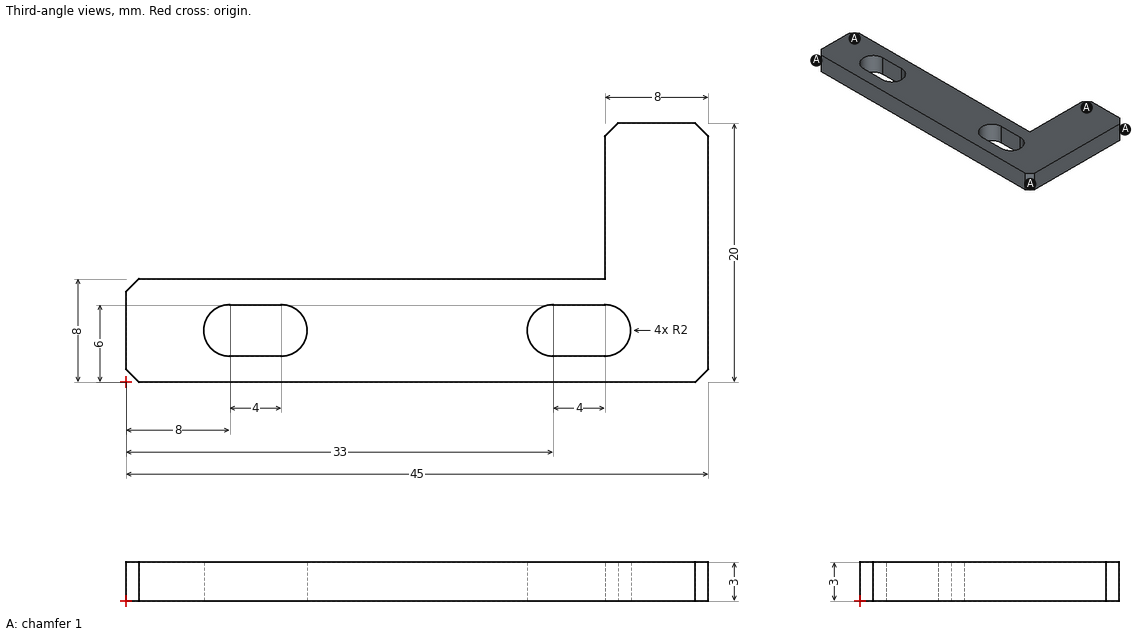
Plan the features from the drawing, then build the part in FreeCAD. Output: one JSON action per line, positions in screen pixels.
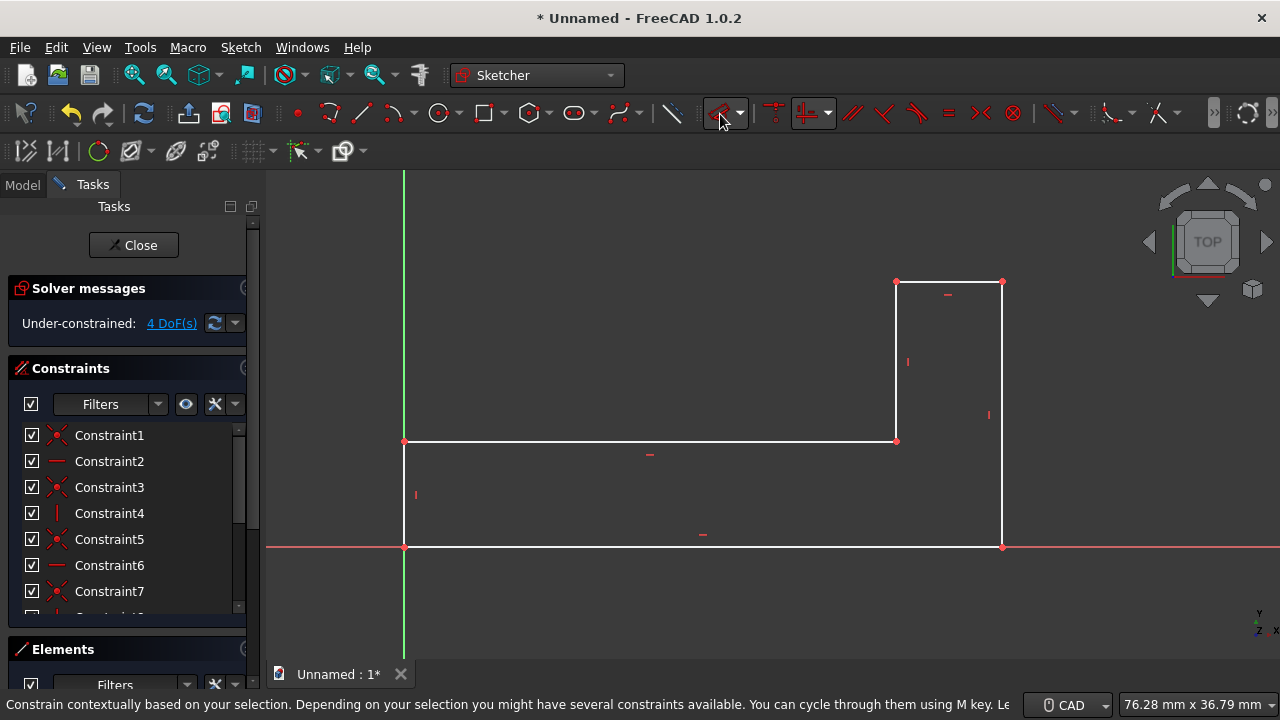
{"action": "left_click", "coordinate": [970, 282]}
{"action": "left_click", "coordinate": [949, 248]}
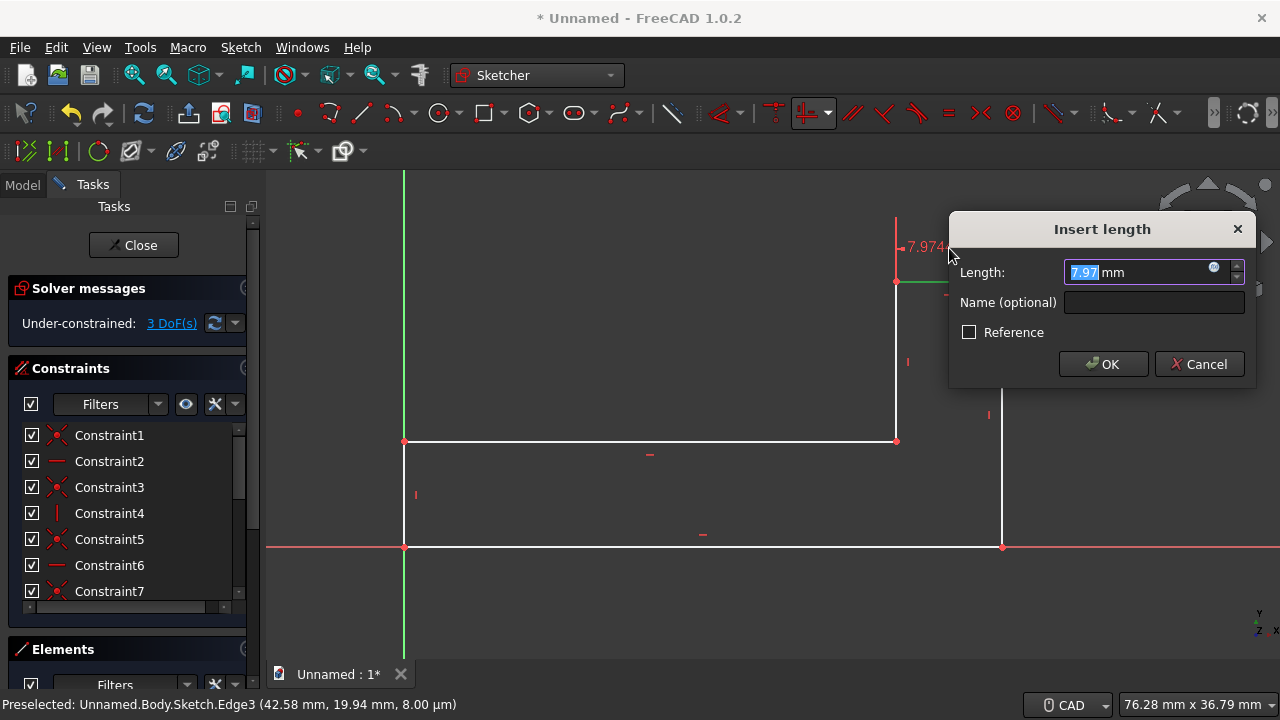
{"action": "type", "text": "8"}
{"action": "key", "text": "Return"}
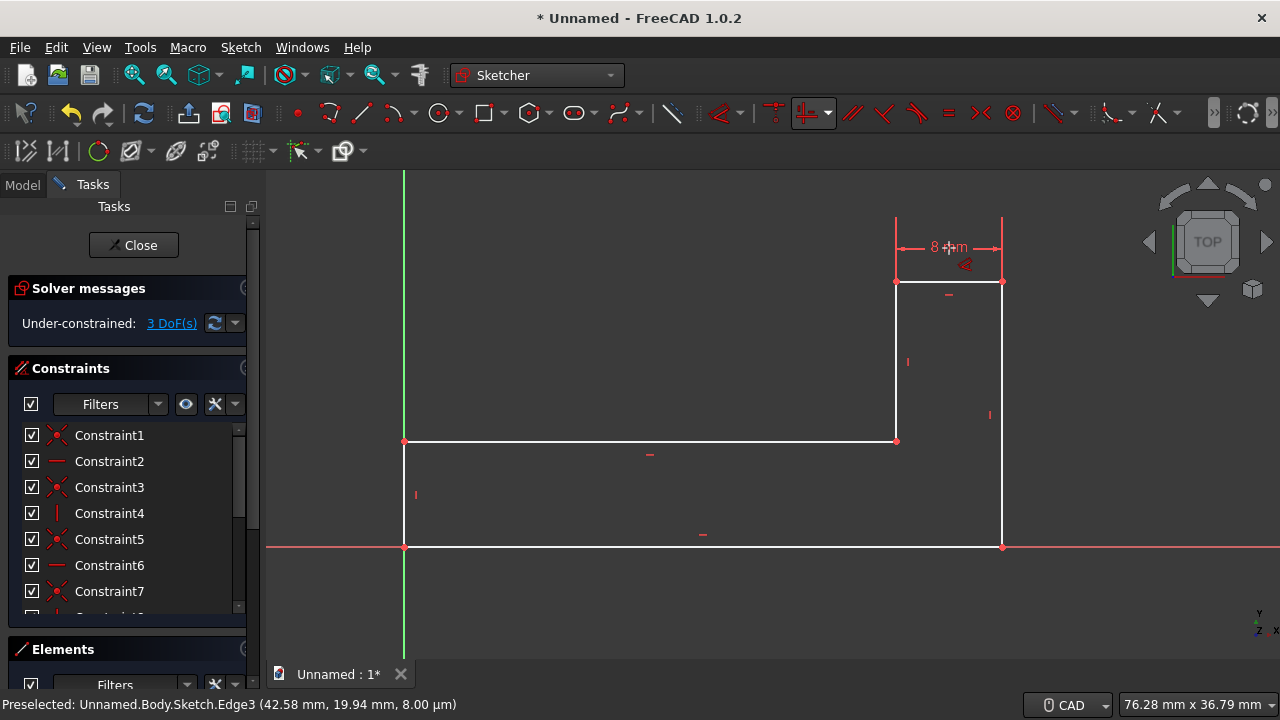
{"action": "left_click", "coordinate": [404, 474]}
{"action": "left_click", "coordinate": [370, 495]}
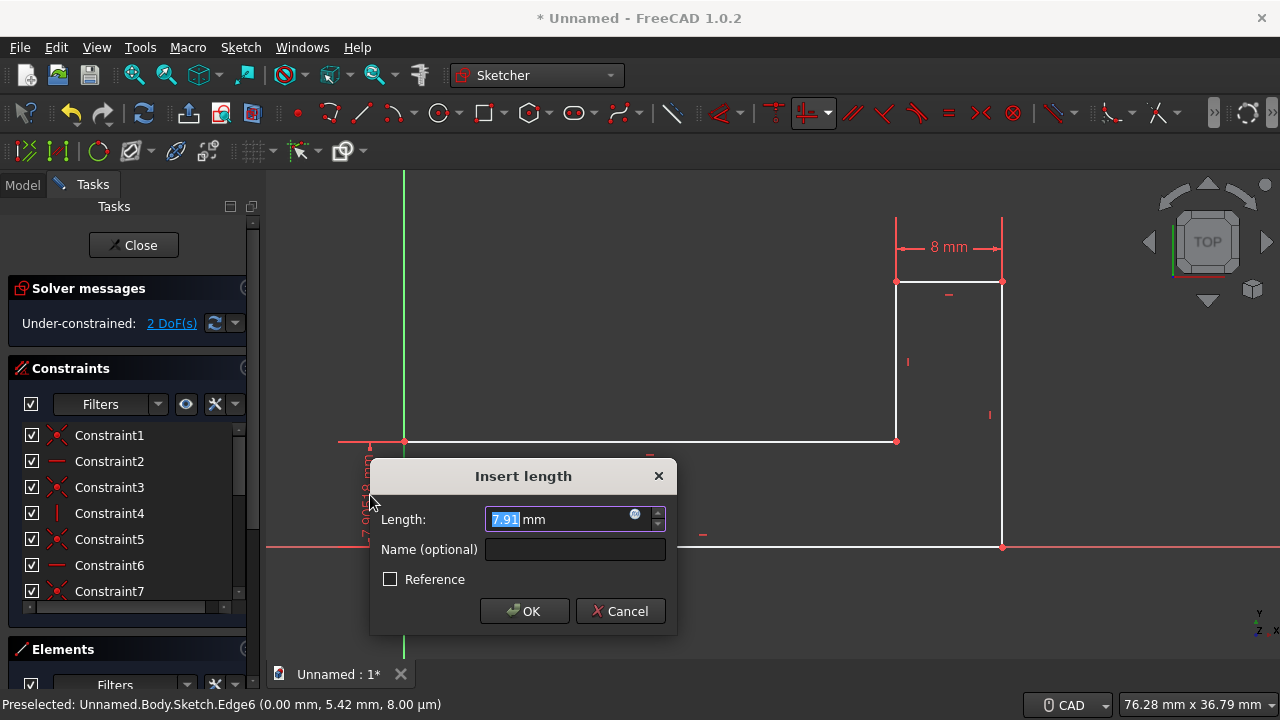
{"action": "type", "text": "8"}
{"action": "key", "text": "Return"}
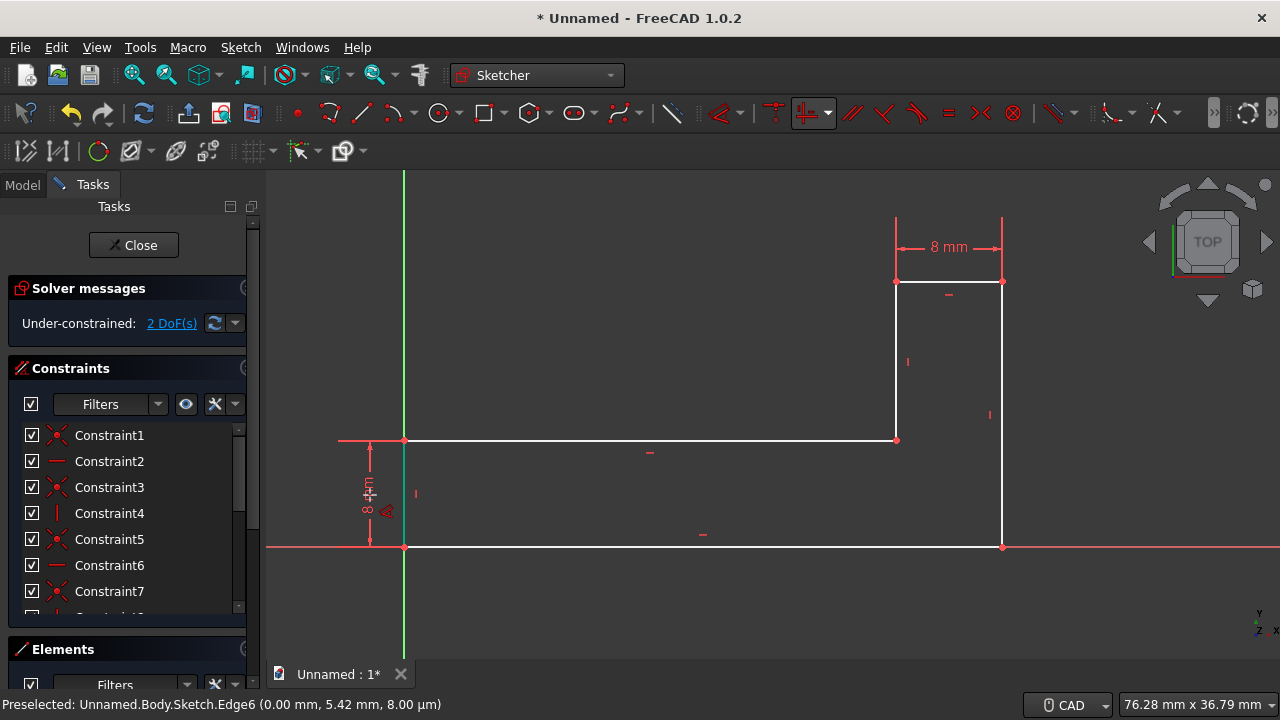
{"action": "left_click", "coordinate": [584, 547]}
{"action": "left_click", "coordinate": [703, 581]}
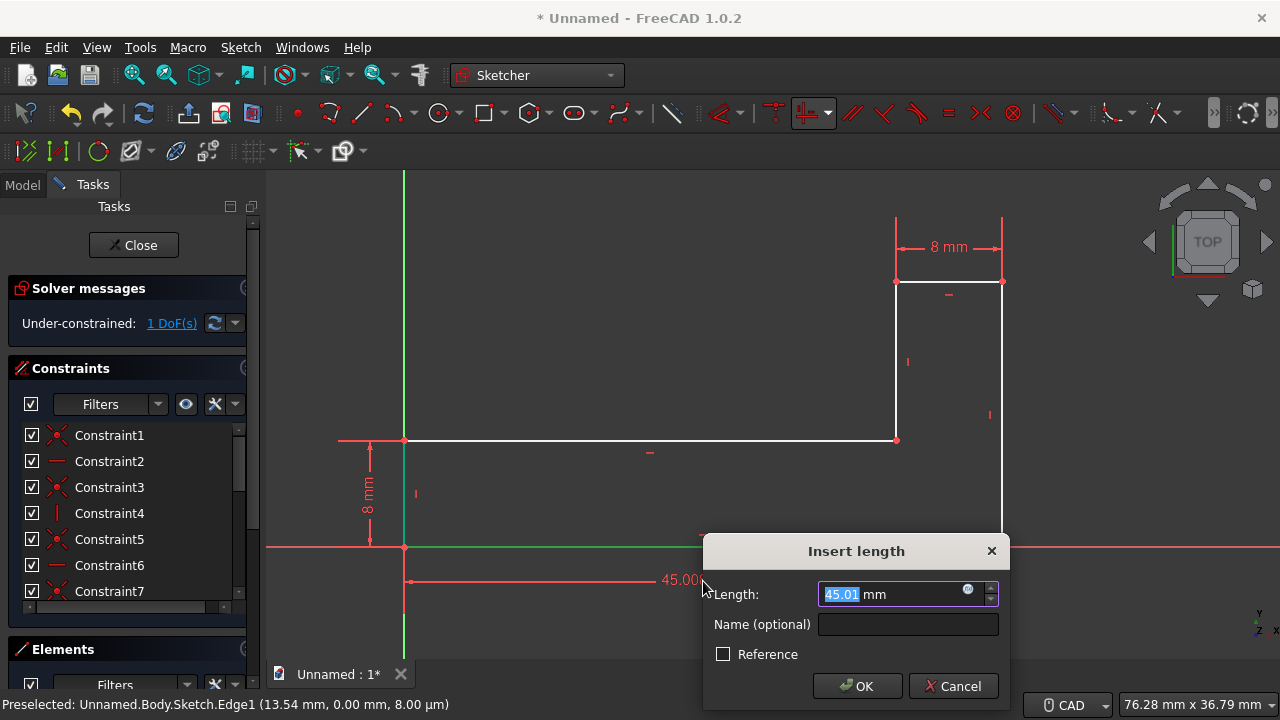
{"action": "type", "text": "45"}
{"action": "key", "text": "Return"}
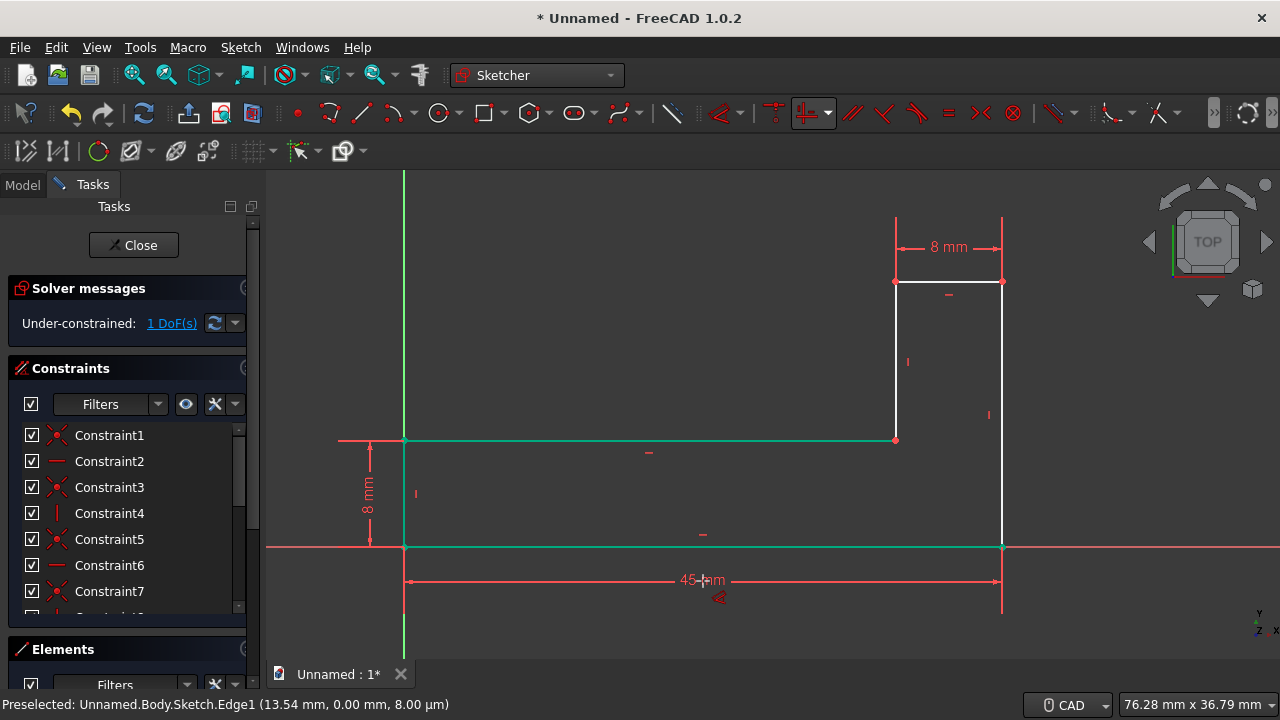
{"action": "left_click", "coordinate": [1002, 468]}
{"action": "left_click", "coordinate": [1036, 415]}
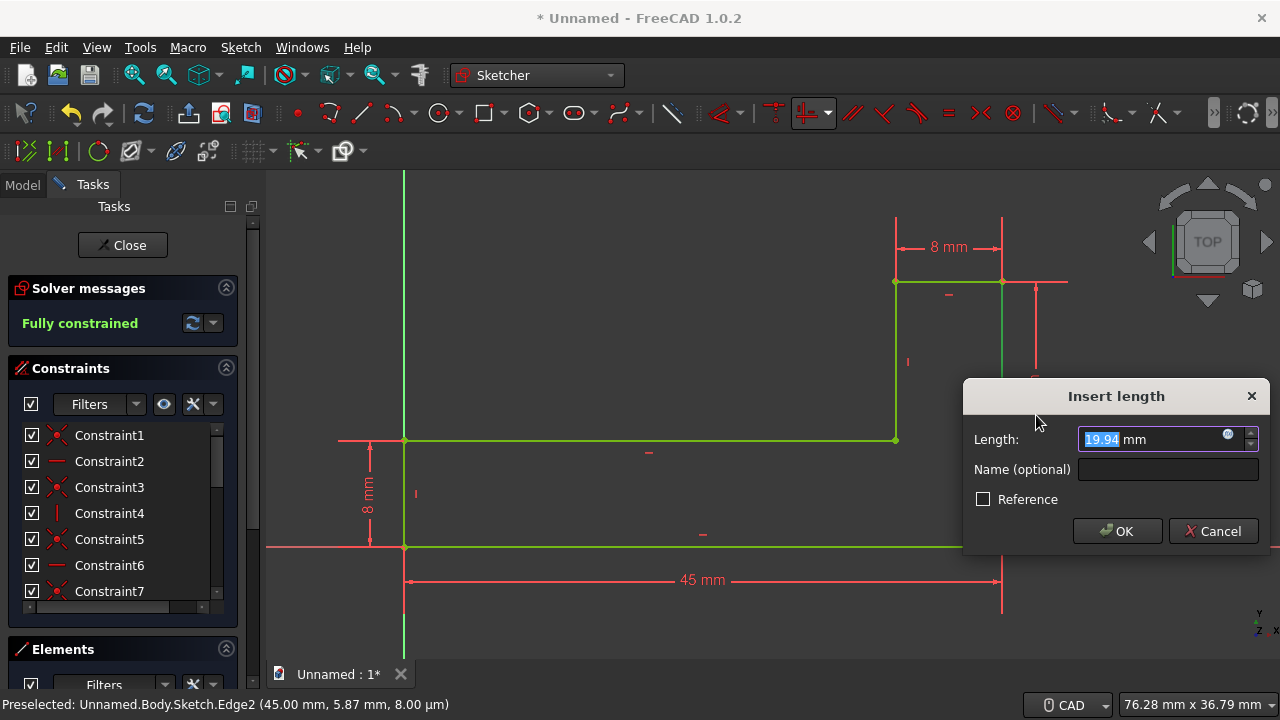
{"action": "type", "text": "20"}
{"action": "key", "text": "Return"}
{"action": "key", "text": "Escape"}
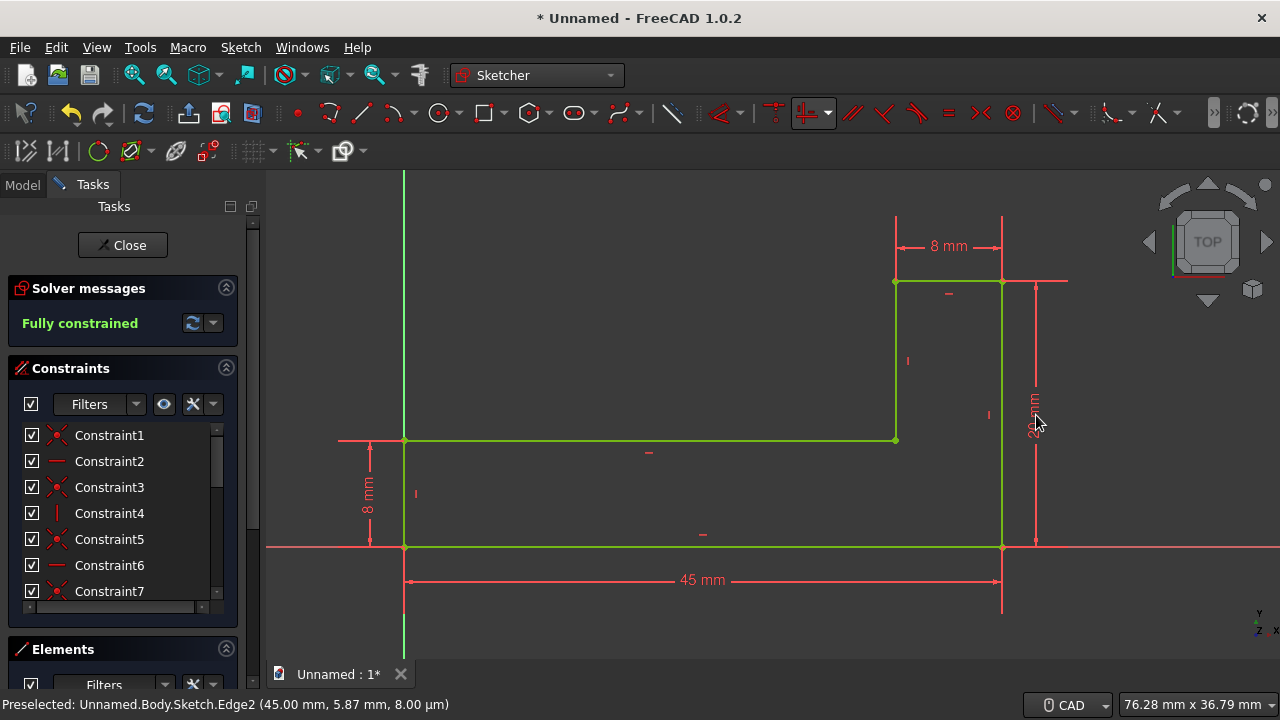
{"action": "left_click", "coordinate": [123, 245]}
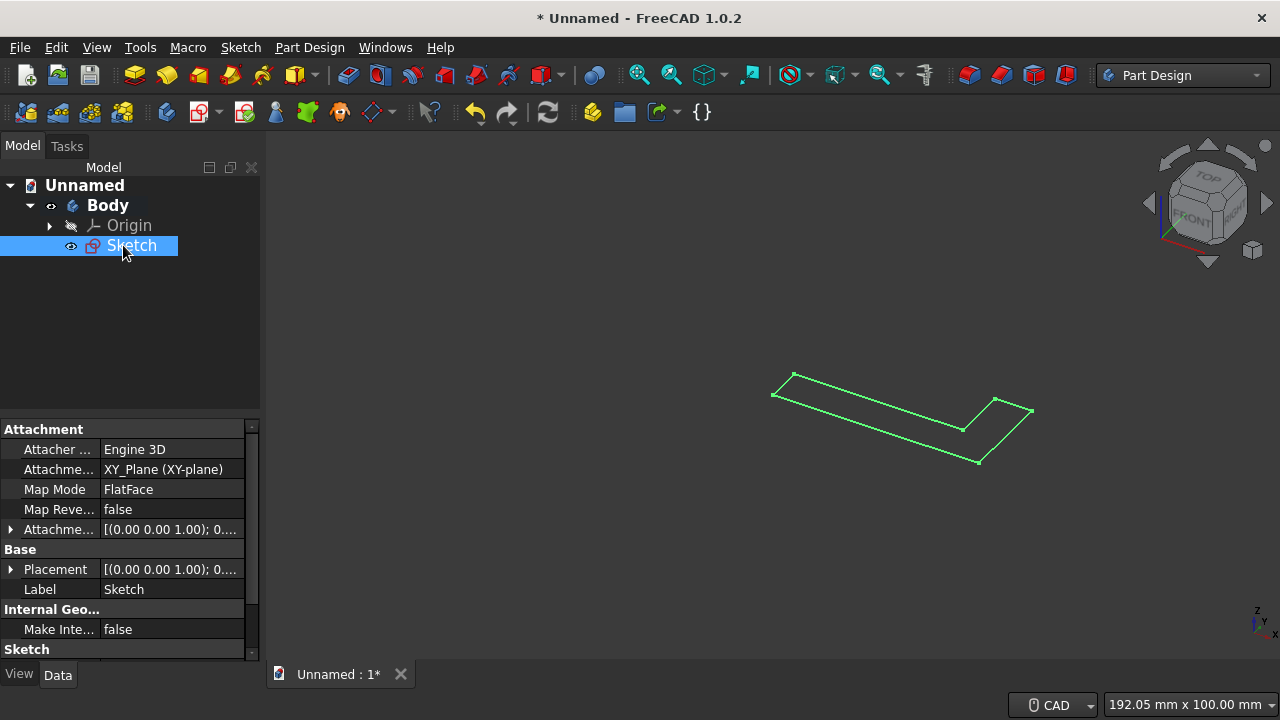
{"action": "left_click", "coordinate": [136, 76]}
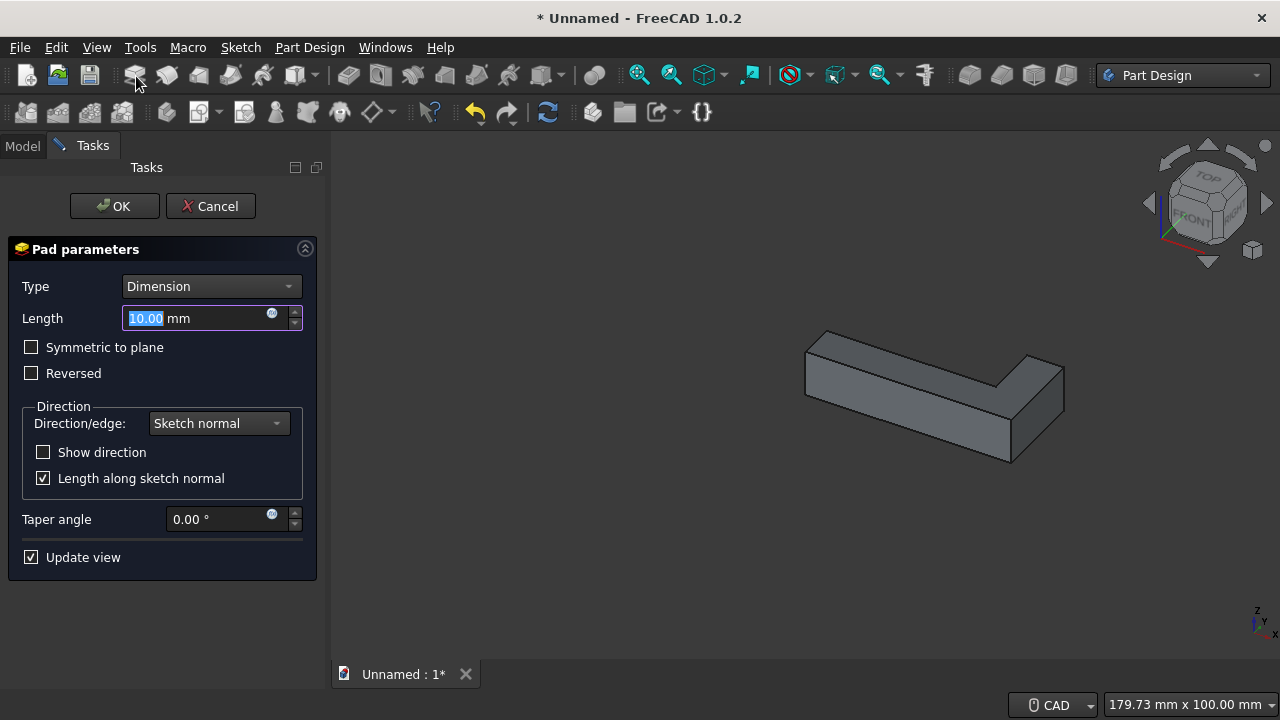
{"action": "type", "text": "3"}
{"action": "key", "text": "Tab"}